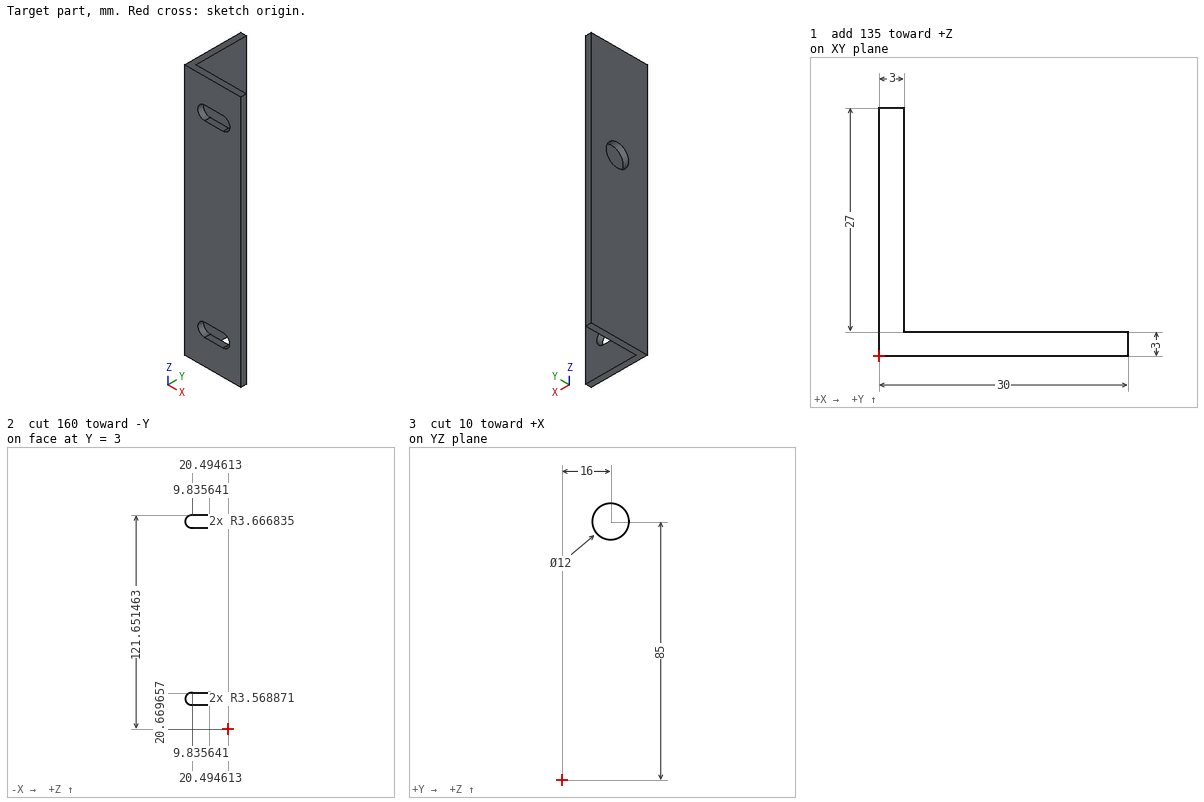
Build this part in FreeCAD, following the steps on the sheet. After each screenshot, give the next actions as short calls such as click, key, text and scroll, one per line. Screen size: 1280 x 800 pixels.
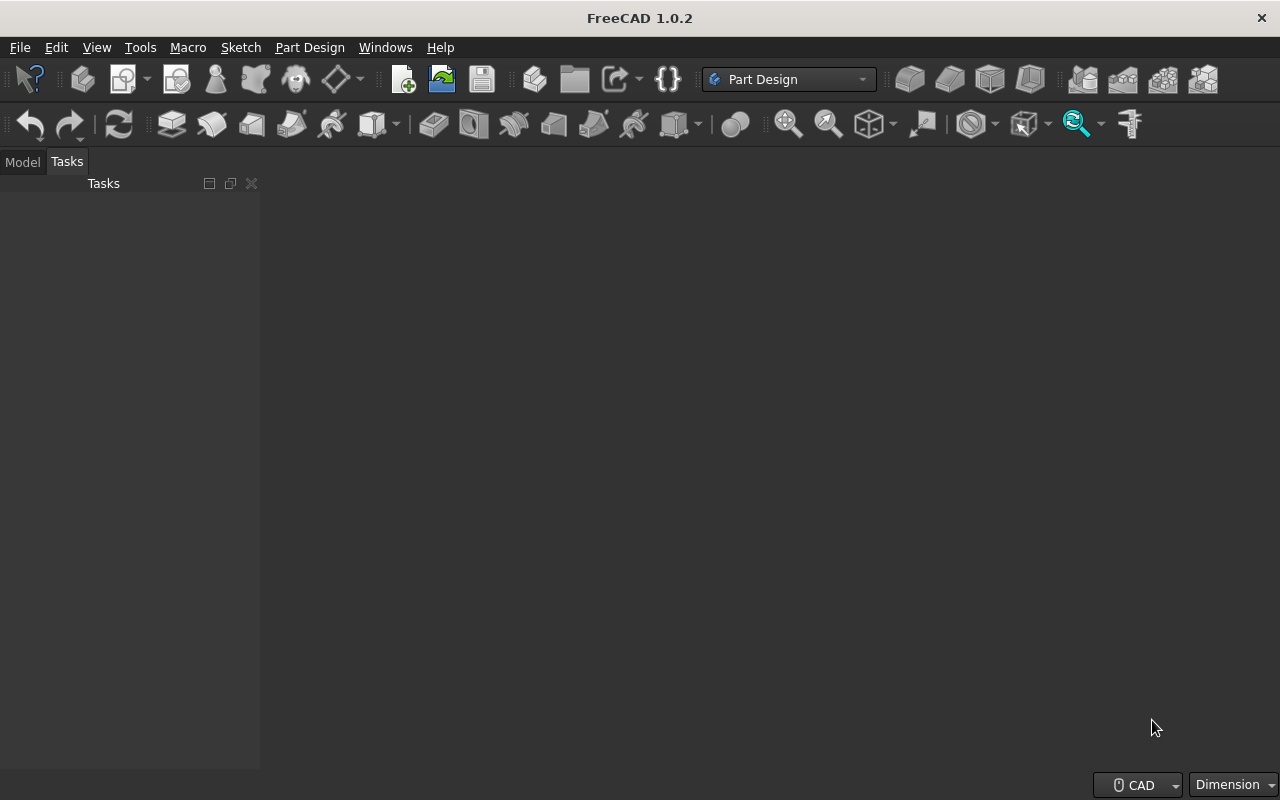
key(ctrl+n)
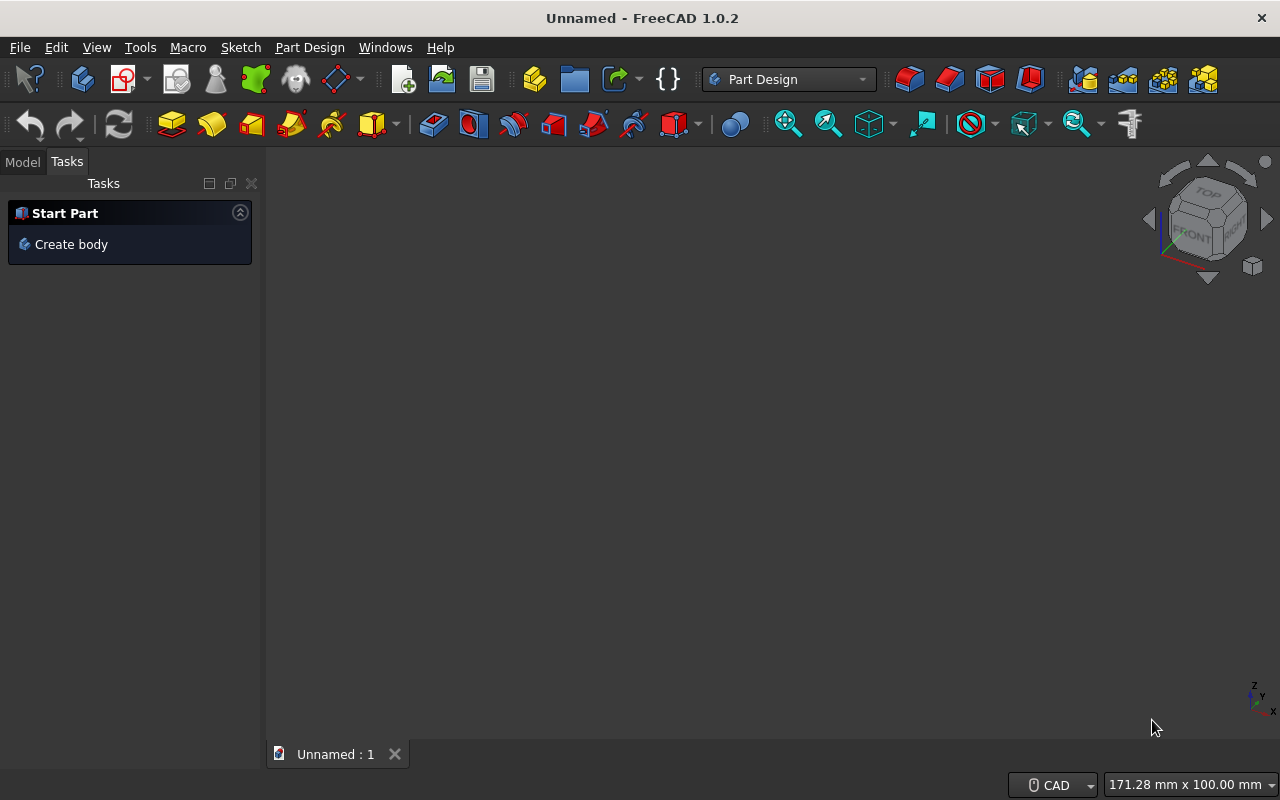
click(124, 80)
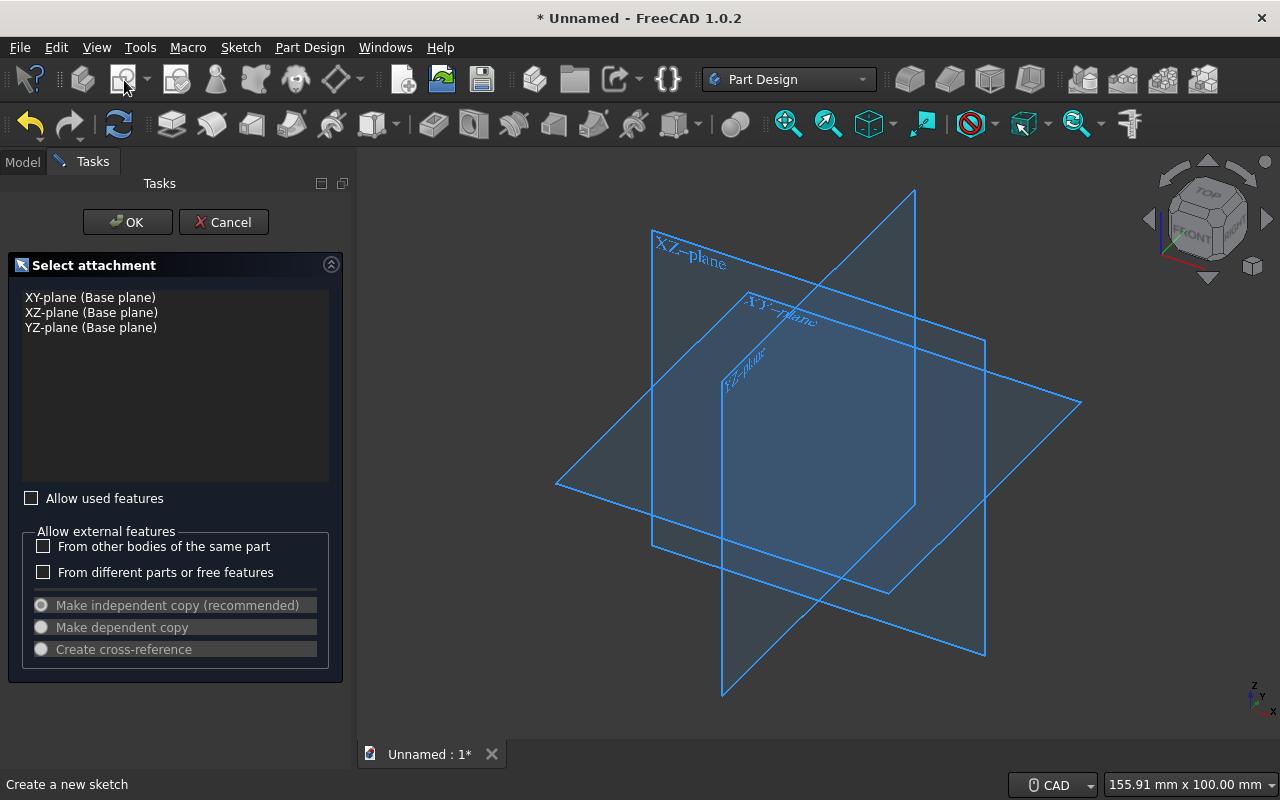
click(82, 298)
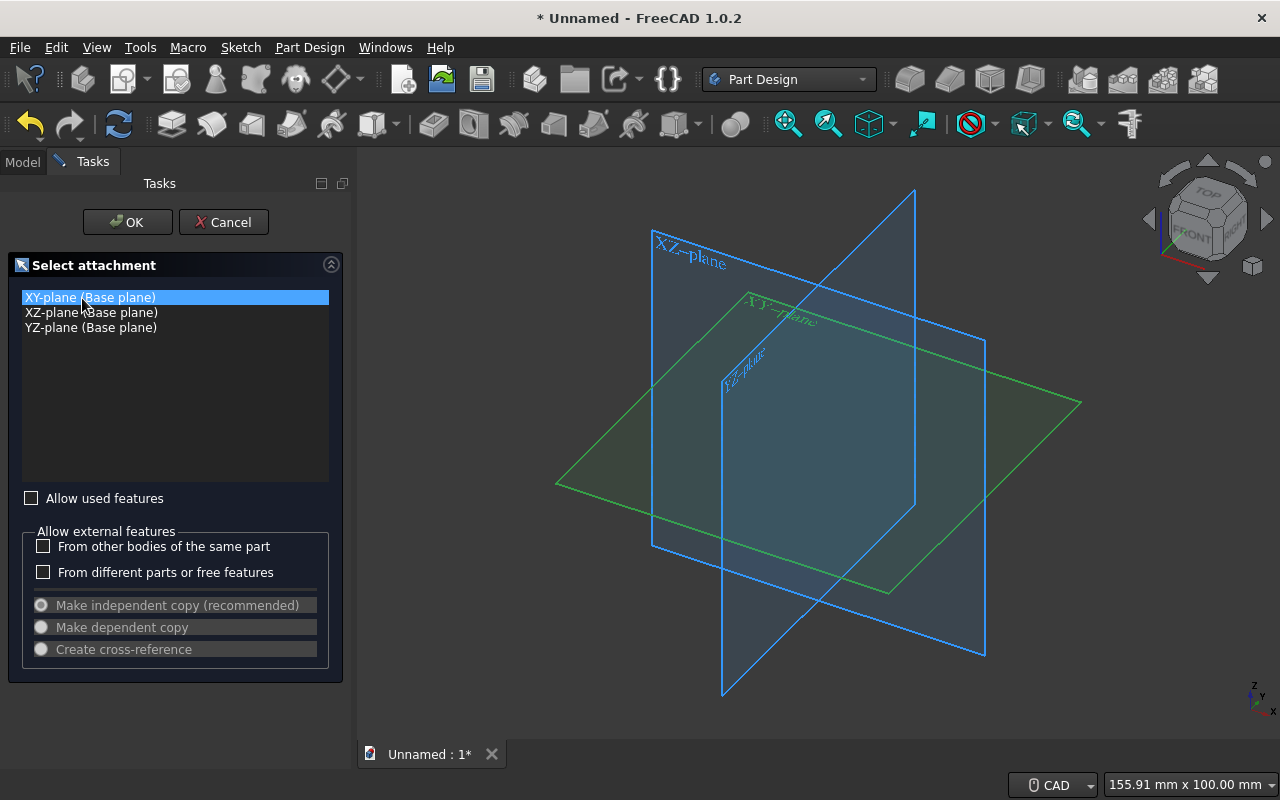
click(128, 222)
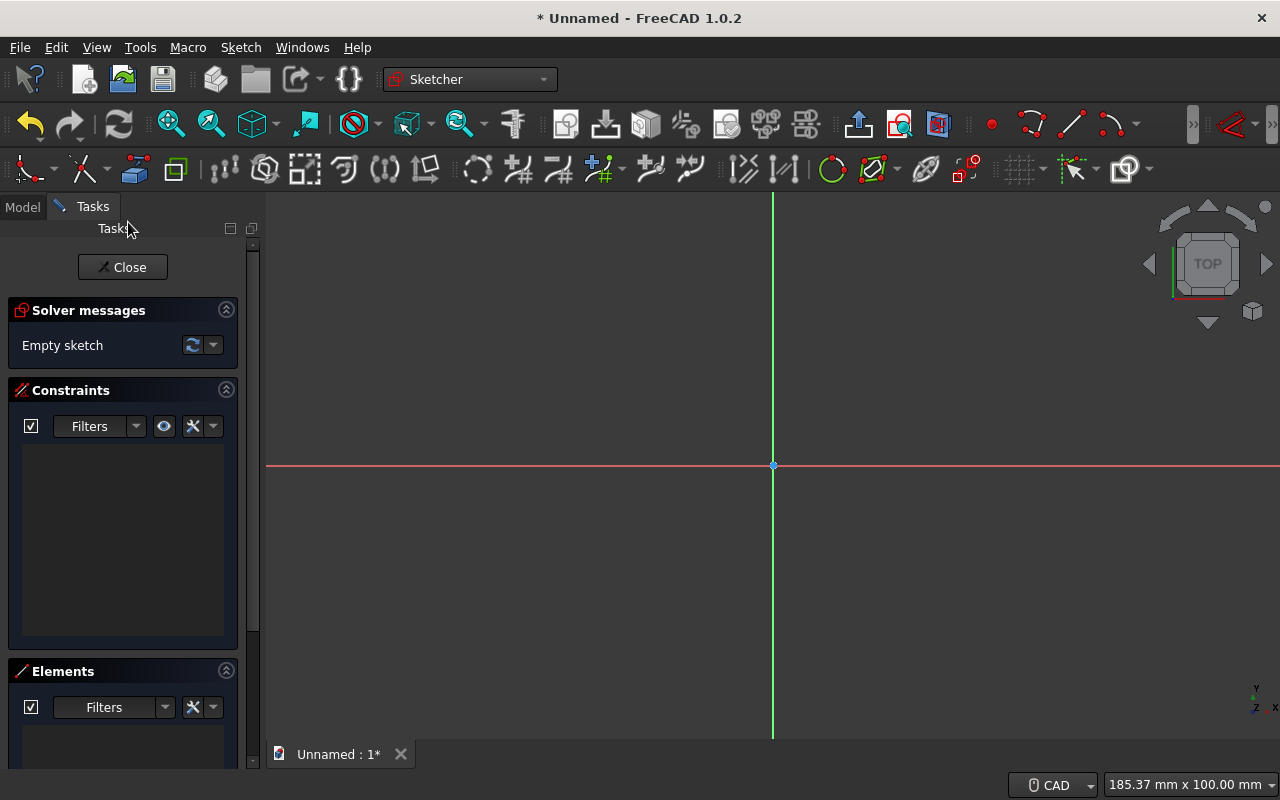
scroll(978, 316, up, 4)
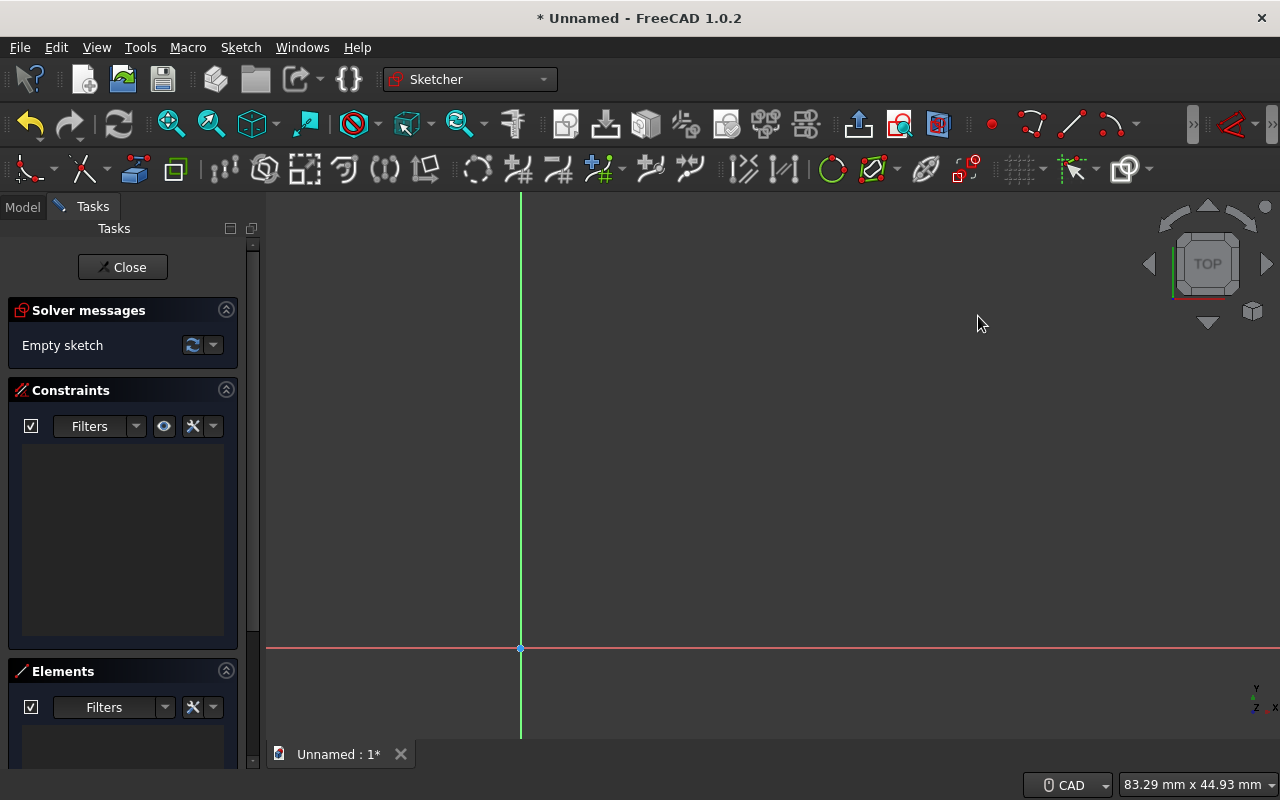
key(g)
key(m)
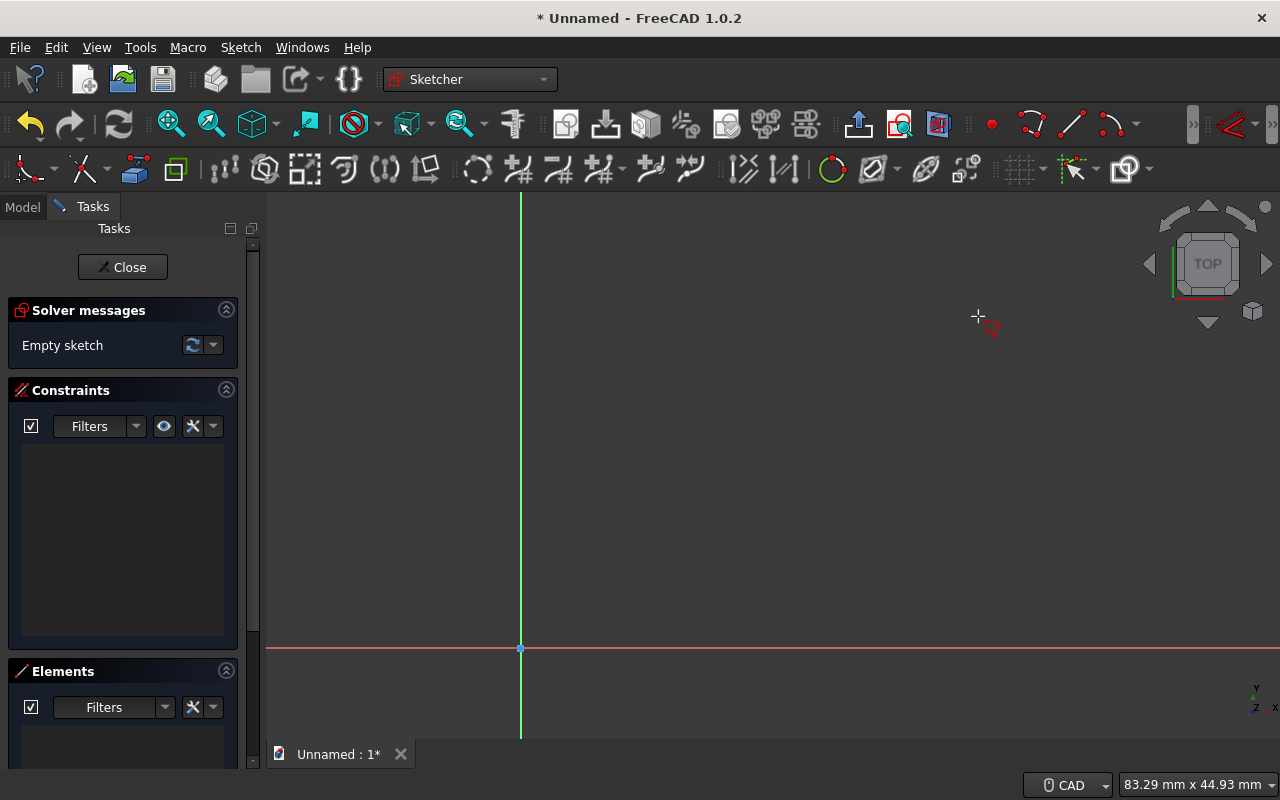
click(521, 648)
click(886, 639)
click(886, 612)
click(557, 612)
click(557, 283)
click(530, 283)
click(521, 648)
key(Escape)
key(Escape)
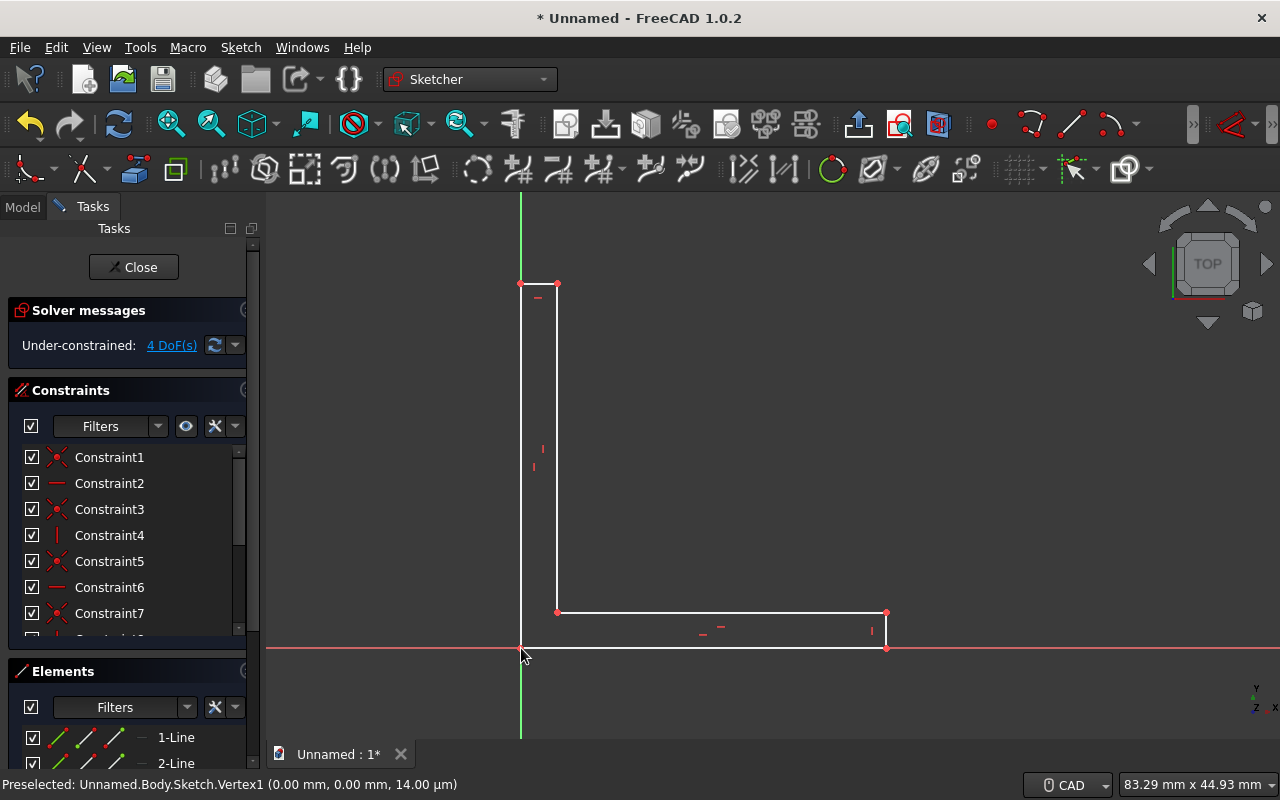
scroll(886, 638, up, 2)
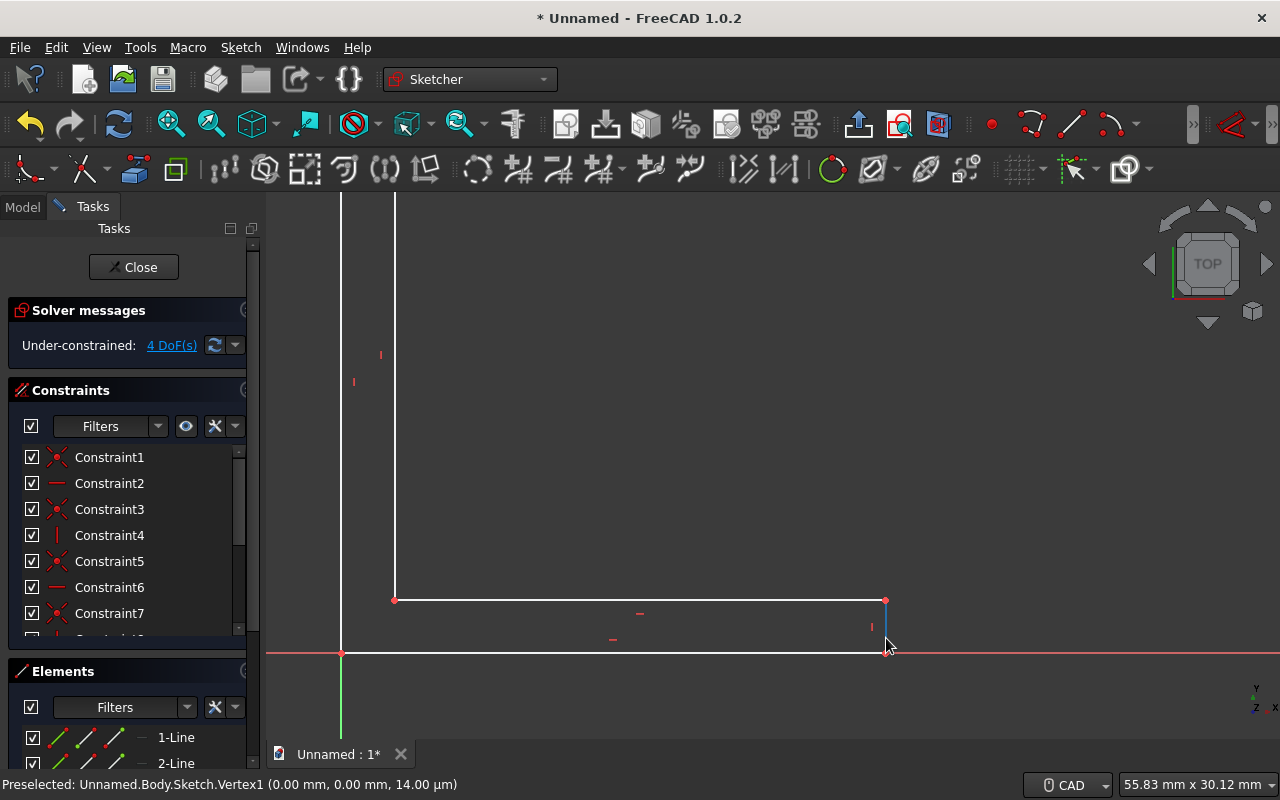
click(886, 637)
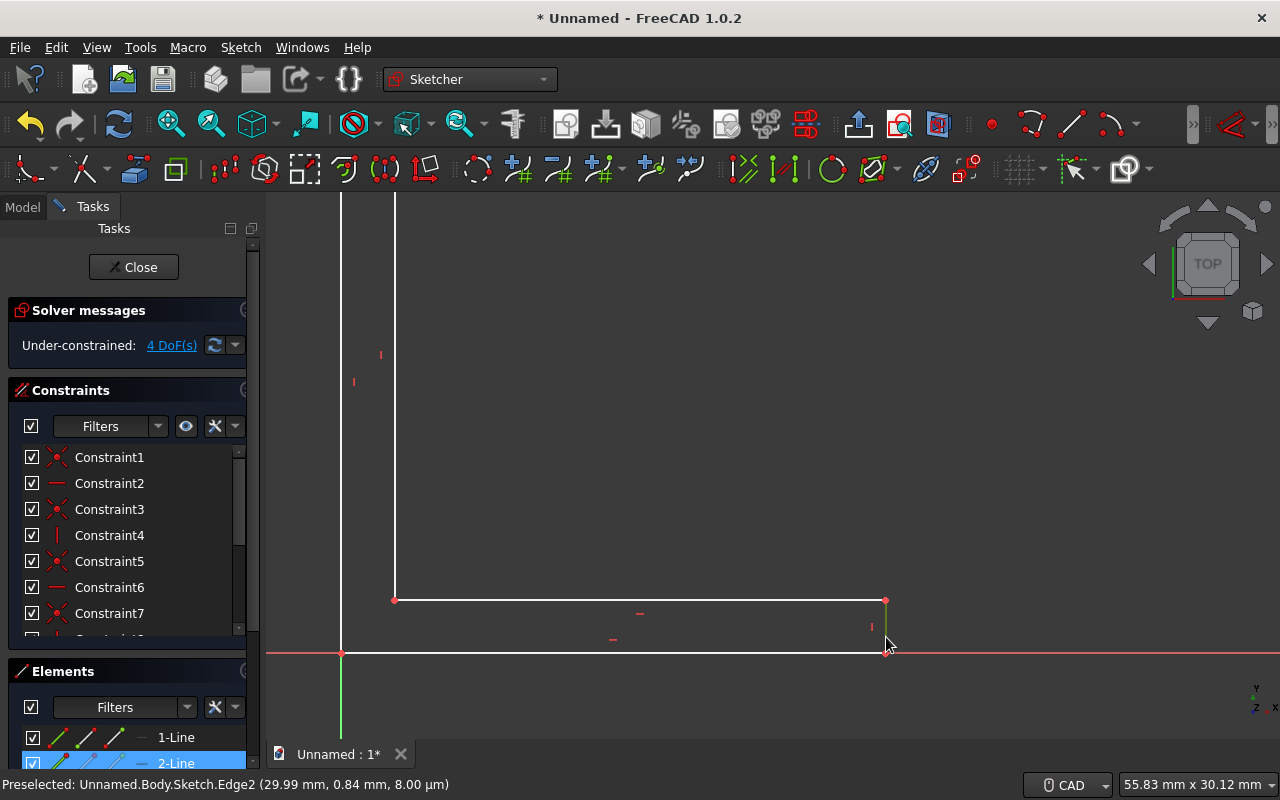
key(i)